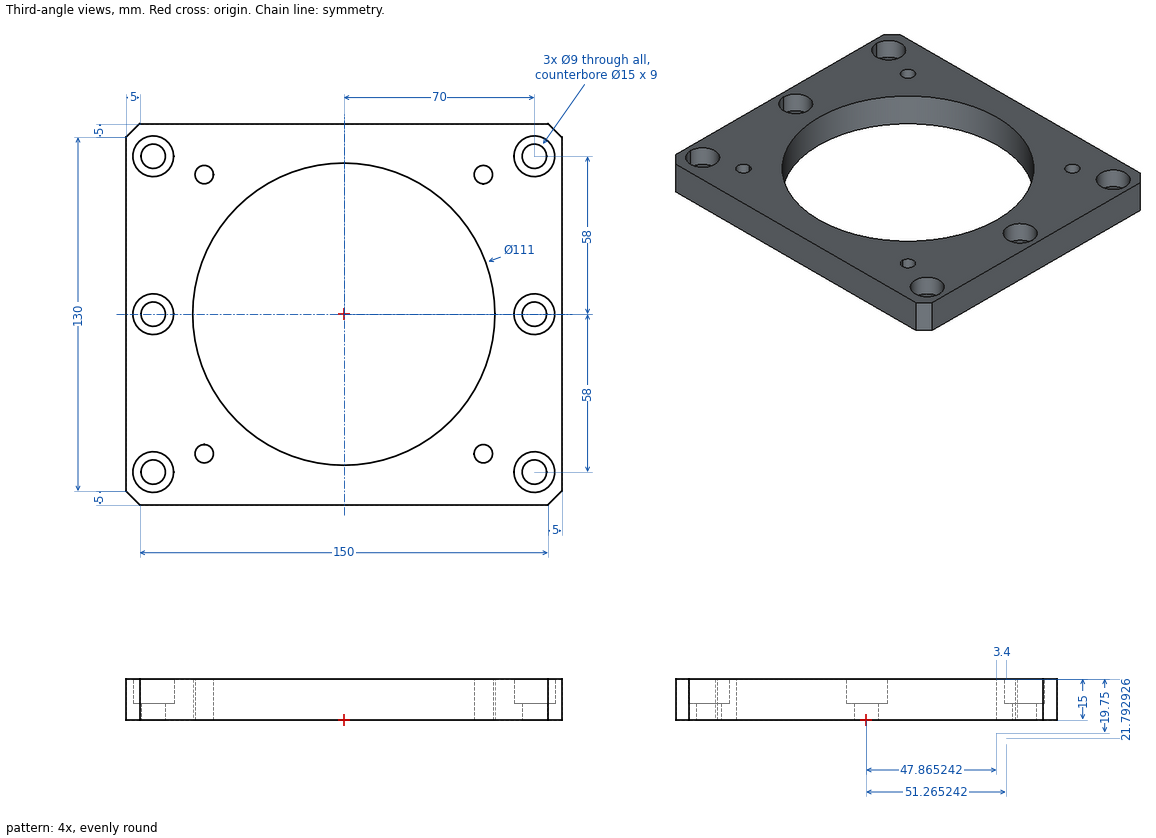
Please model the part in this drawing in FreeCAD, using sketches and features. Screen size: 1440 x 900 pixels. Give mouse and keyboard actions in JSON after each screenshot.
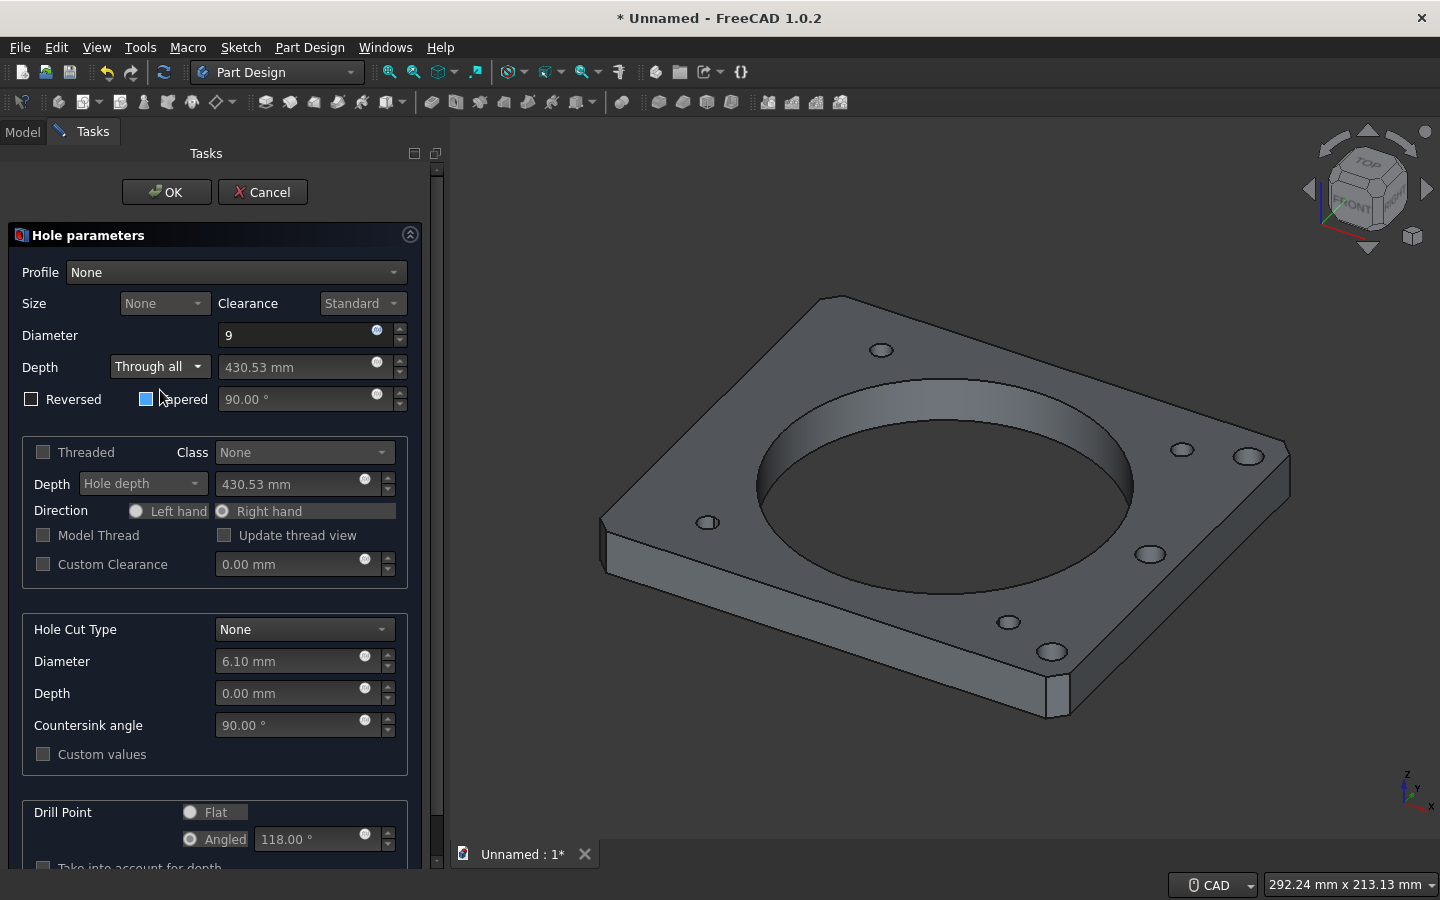
{"action": "left_click", "coordinate": [306, 630]}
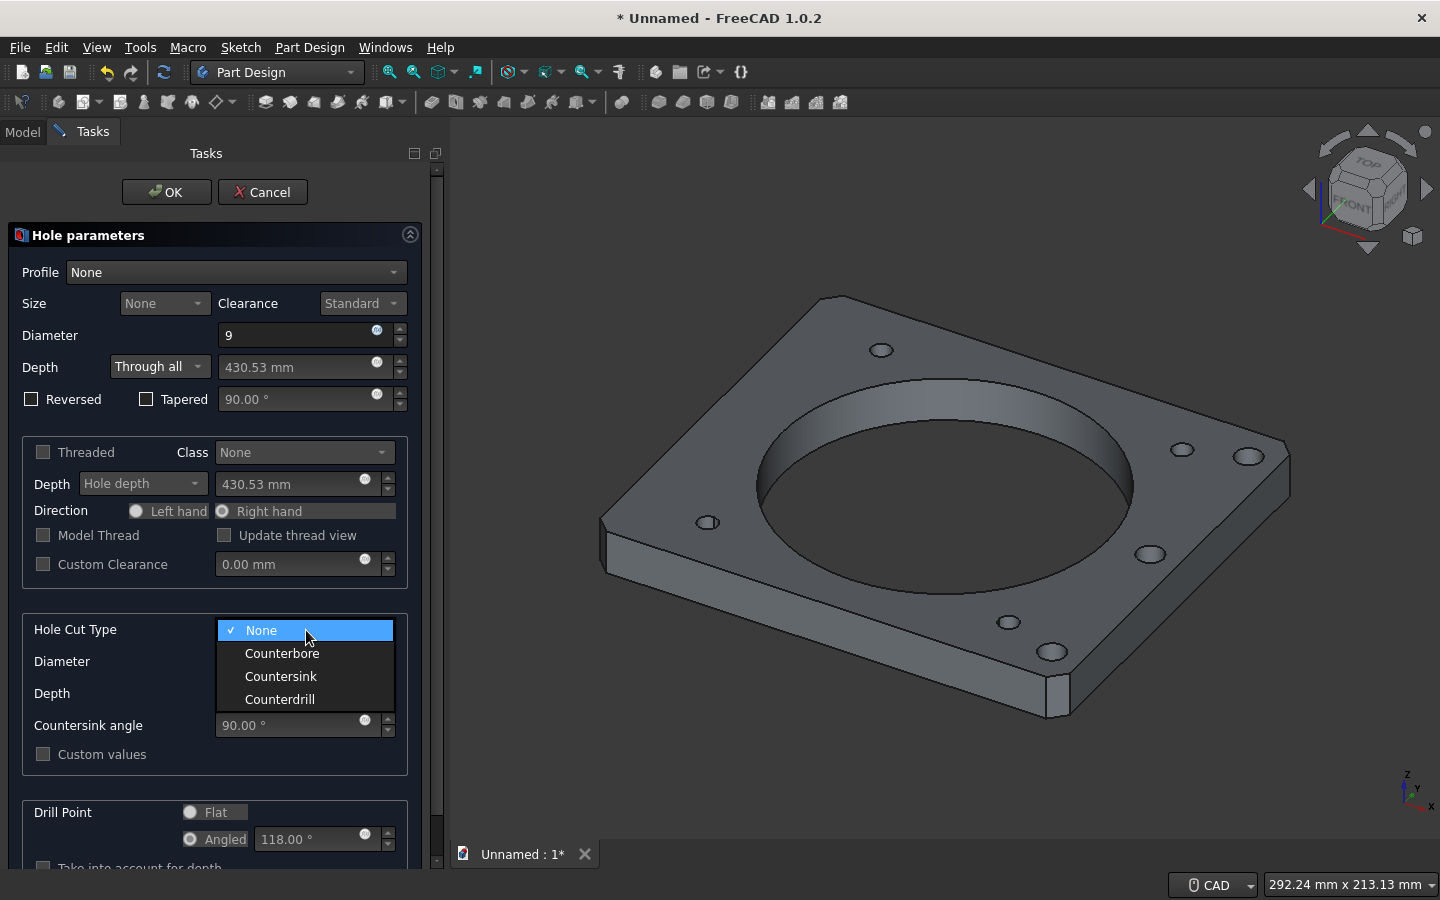
{"action": "left_click", "coordinate": [304, 654]}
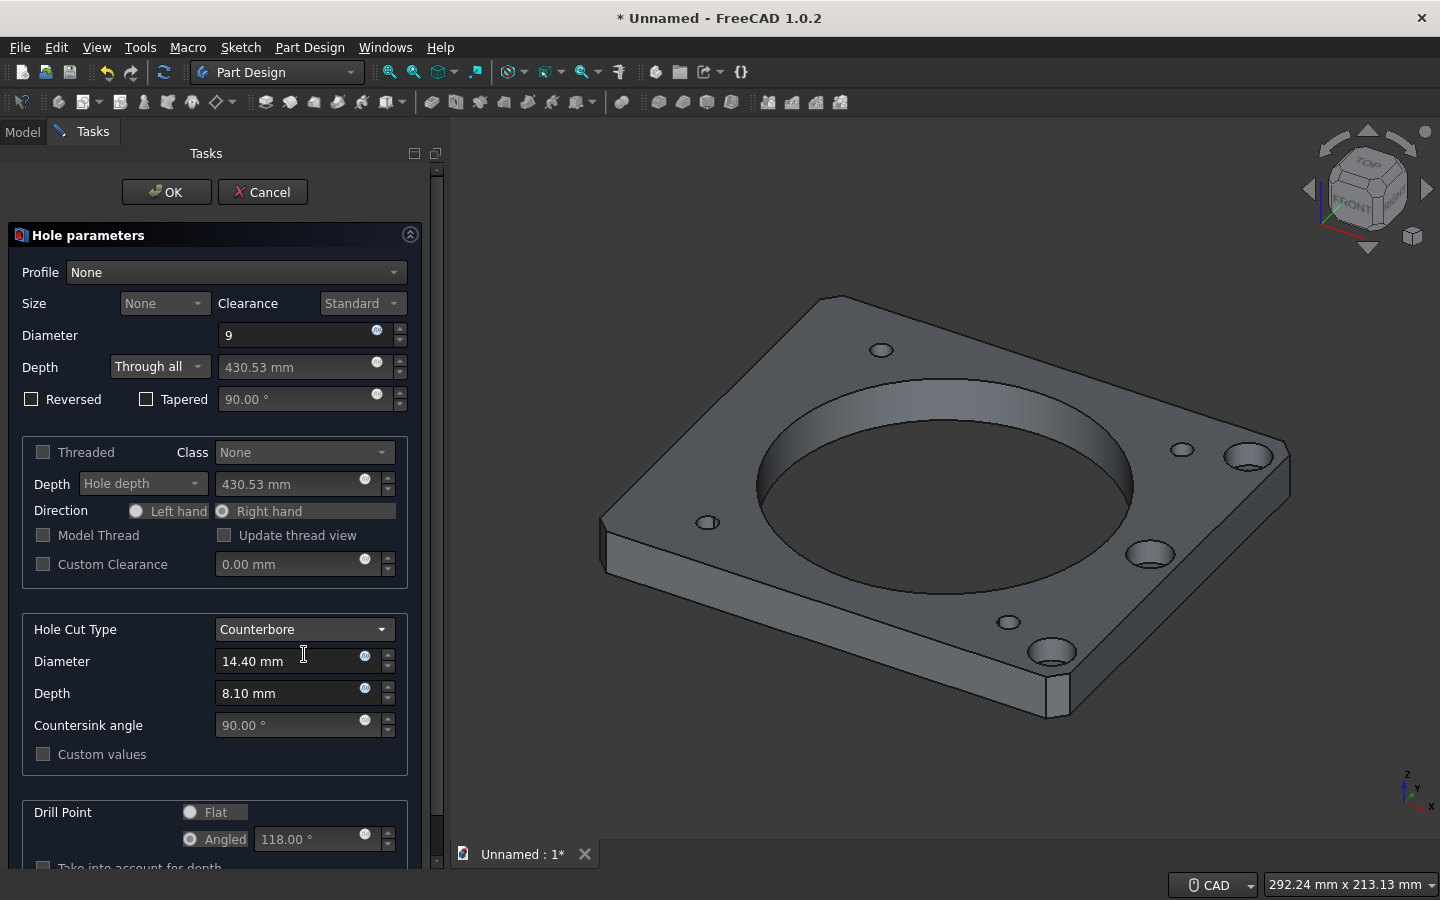
{"action": "triple_click", "coordinate": [298, 661]}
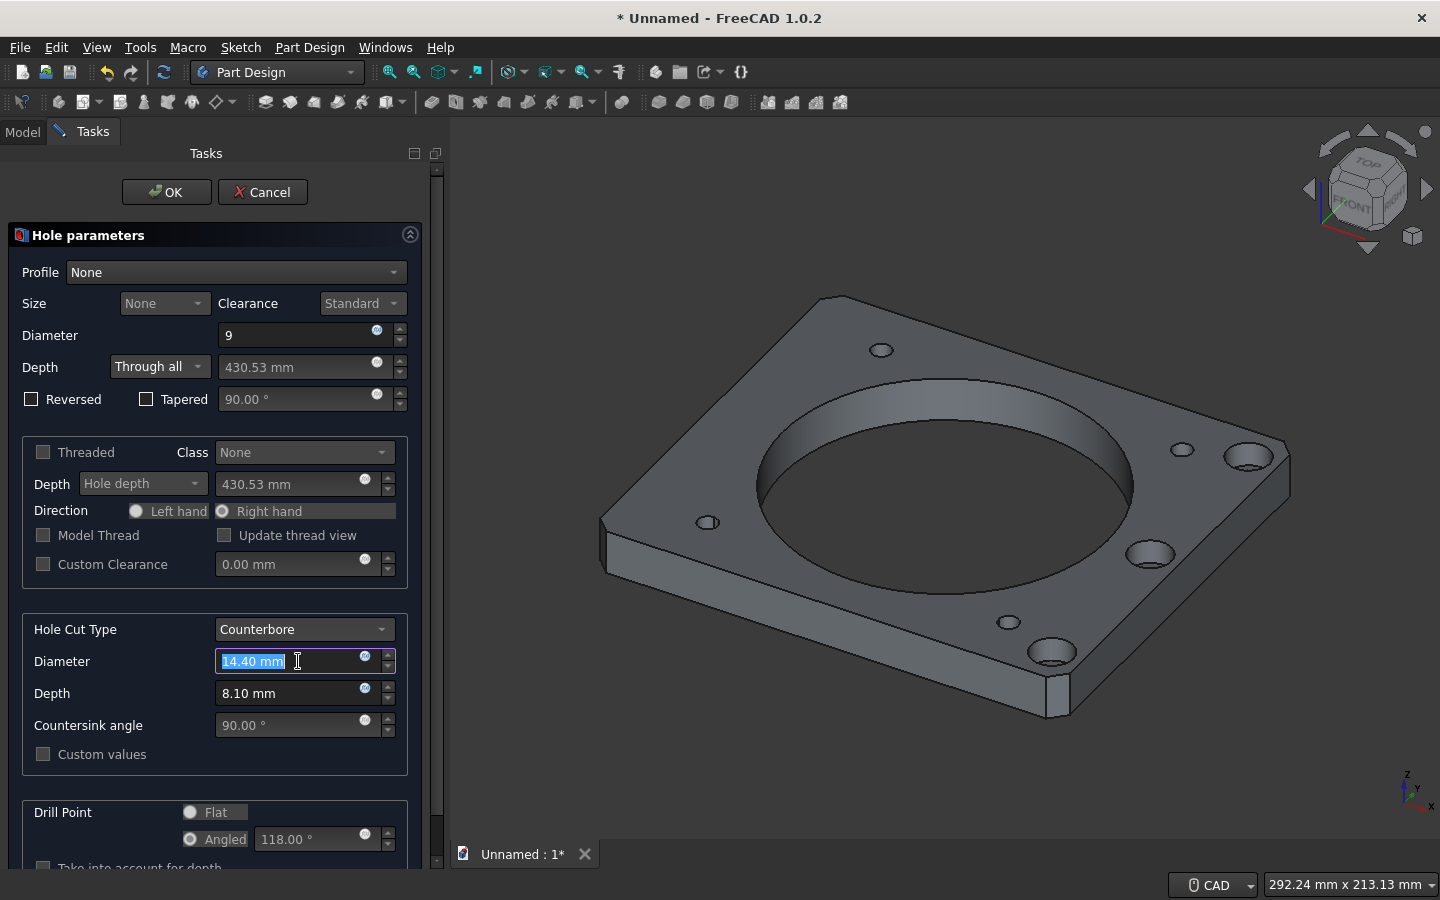
{"action": "type", "text": "15"}
{"action": "key", "text": "Tab"}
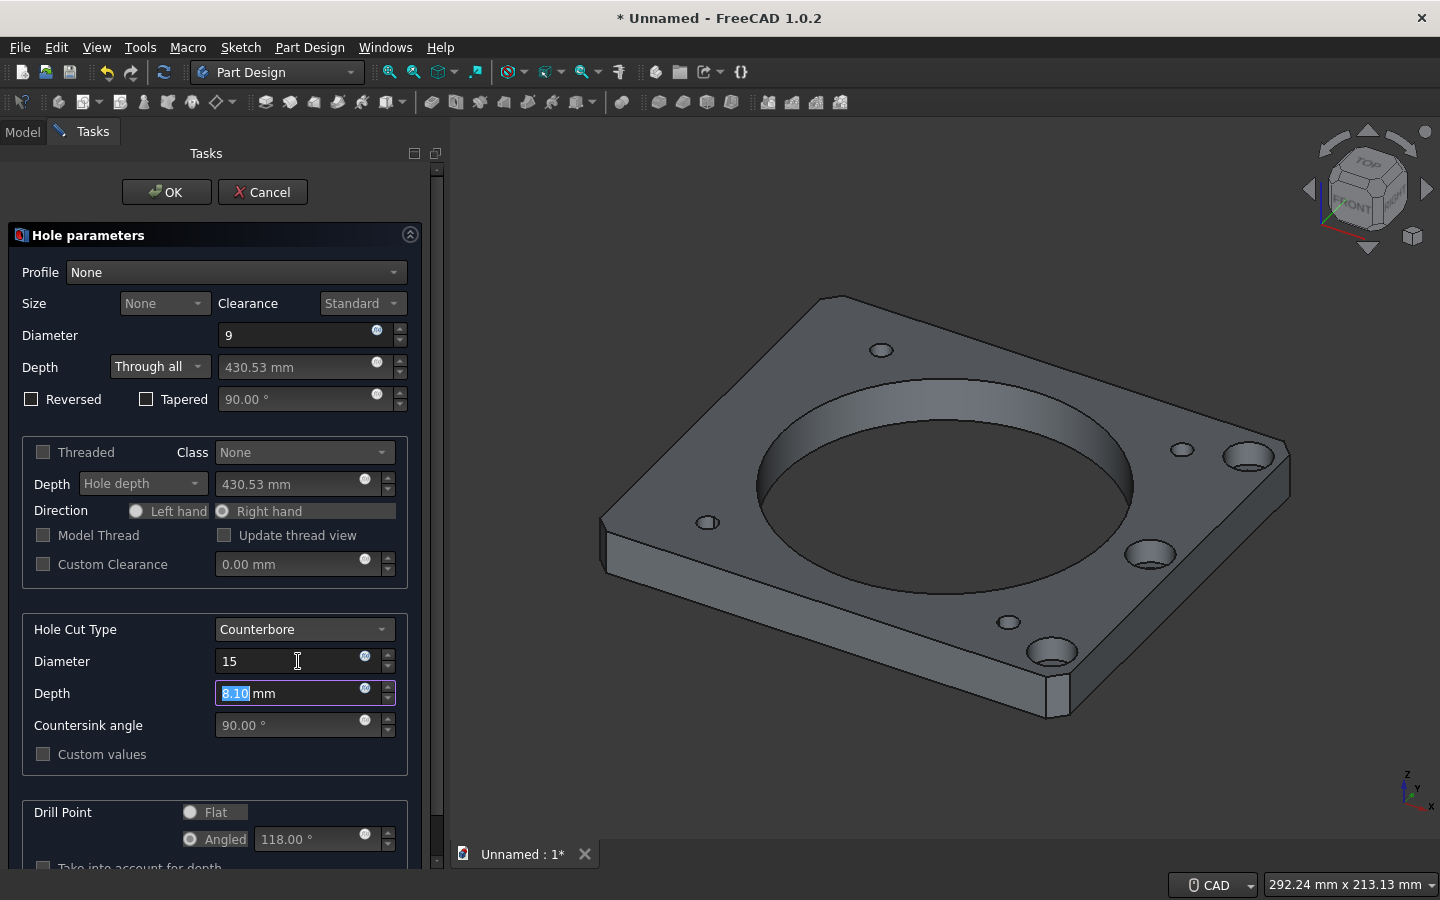
{"action": "type", "text": "9"}
{"action": "key", "text": "Tab"}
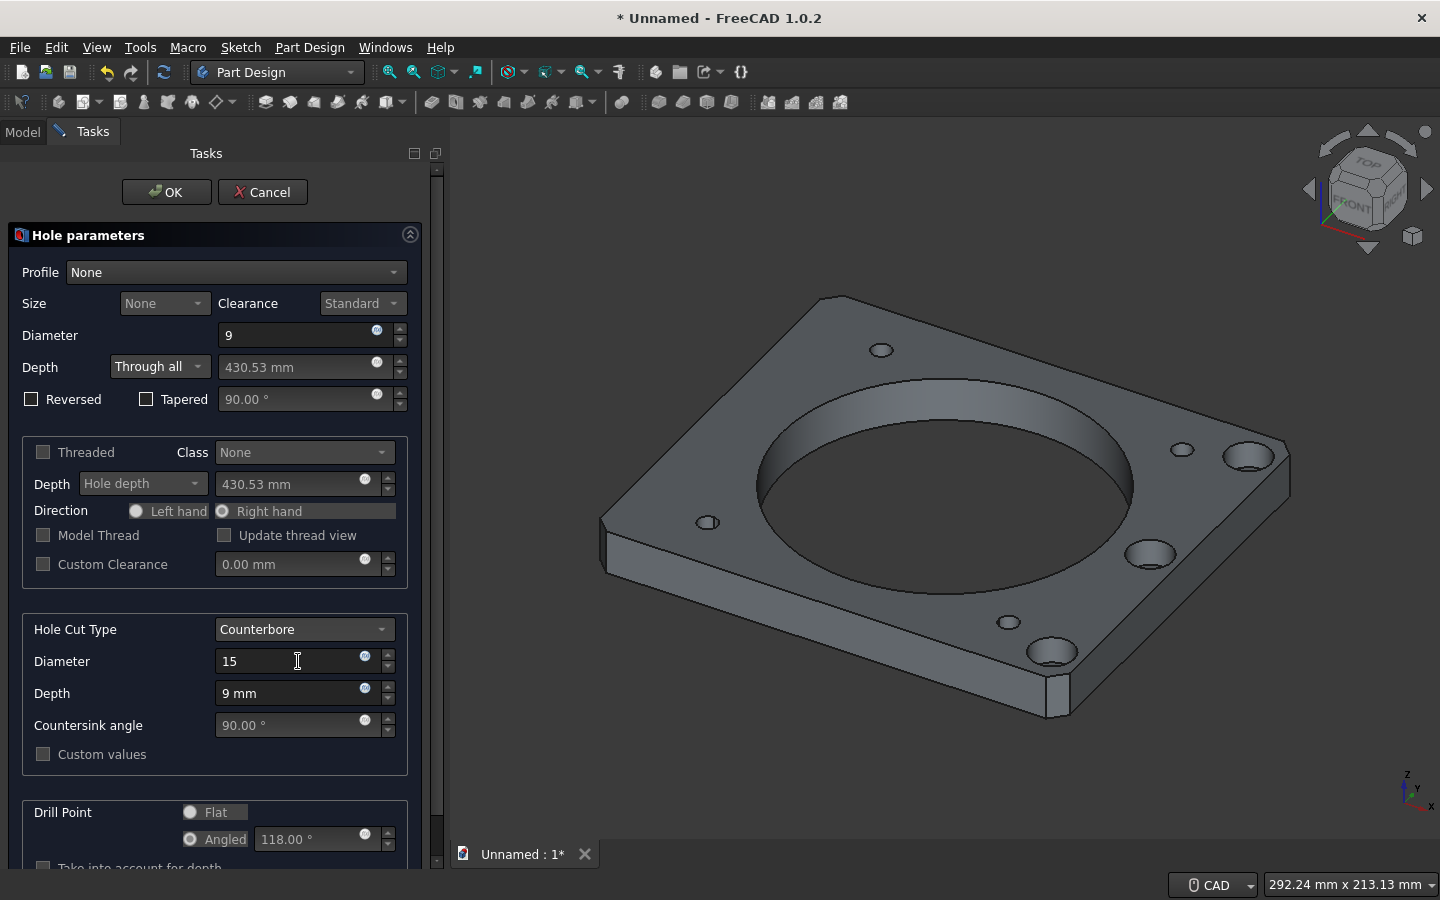
{"action": "left_click", "coordinate": [167, 192]}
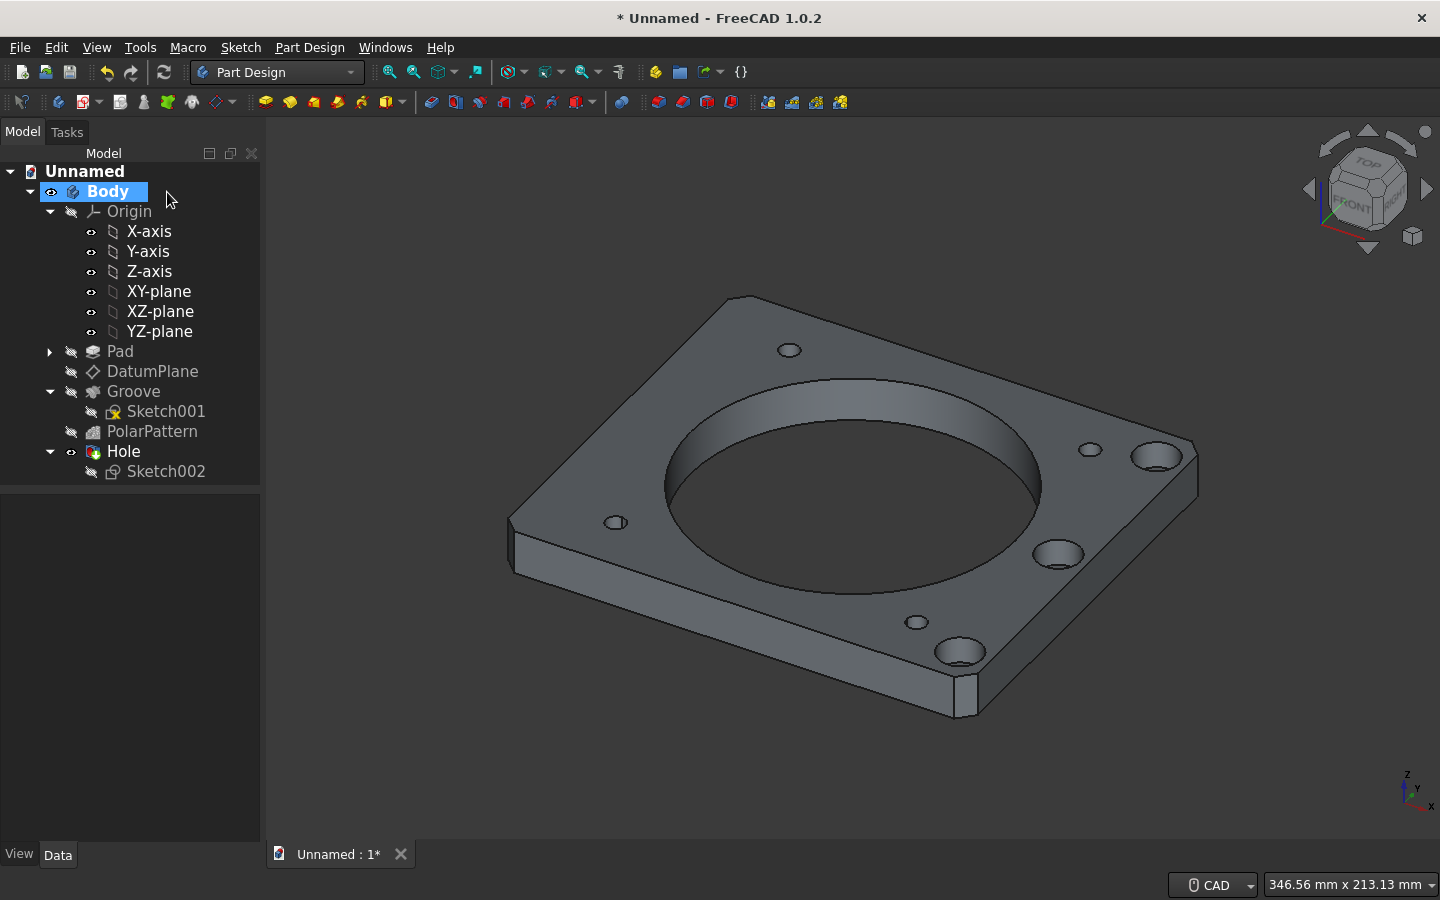
{"action": "left_click", "coordinate": [116, 452]}